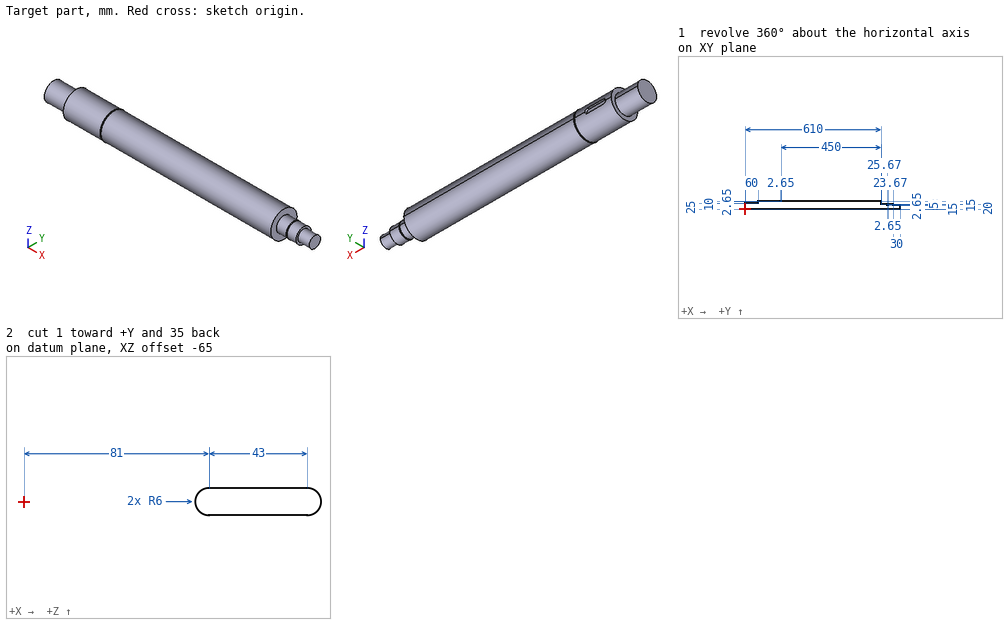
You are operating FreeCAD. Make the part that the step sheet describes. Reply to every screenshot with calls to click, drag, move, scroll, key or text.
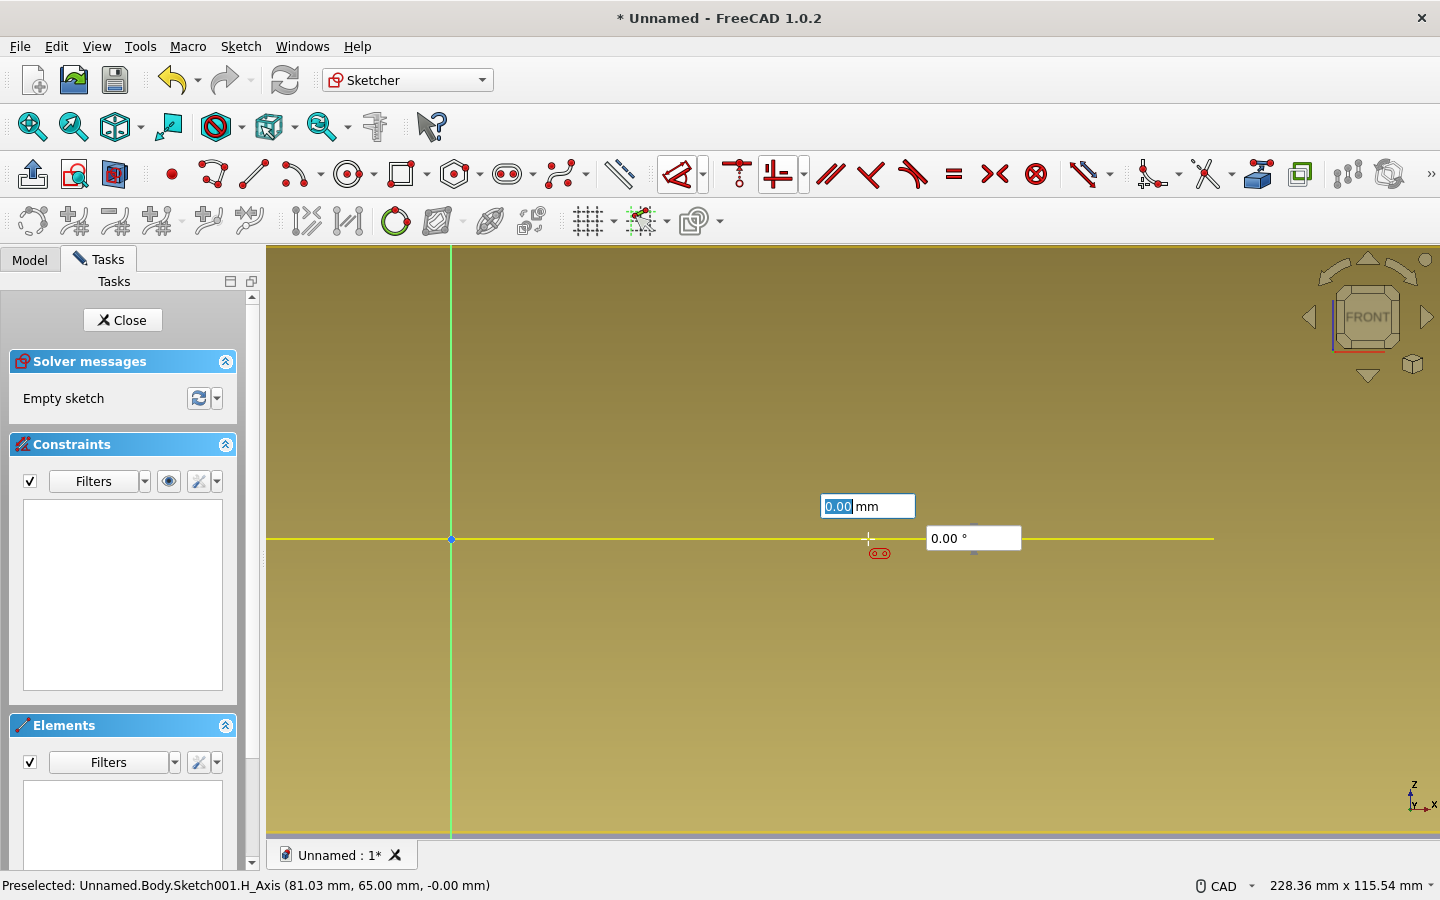
click(1089, 530)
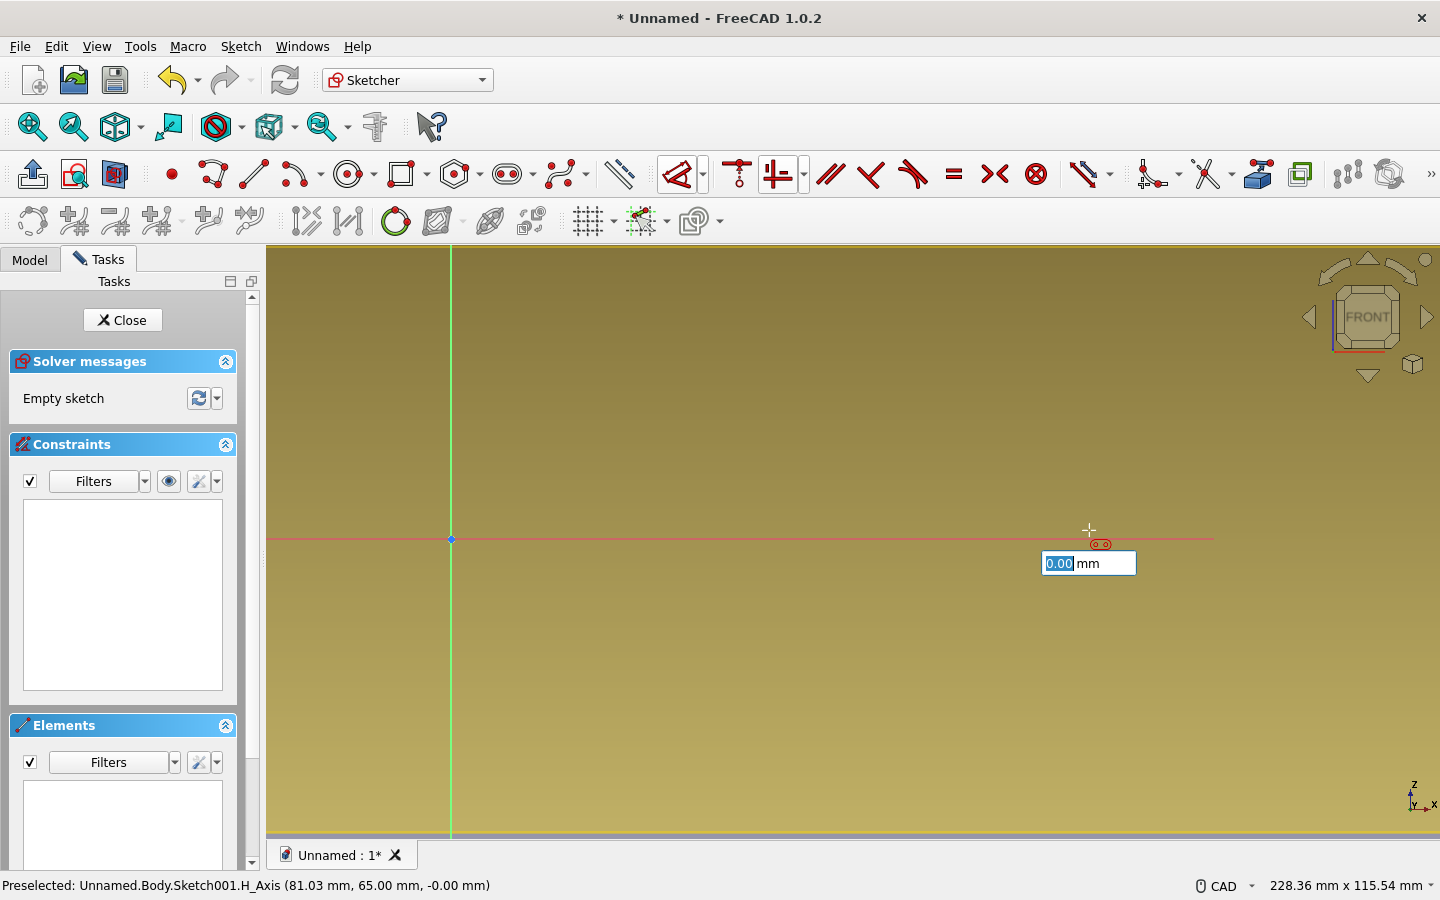
click(978, 570)
key(Escape)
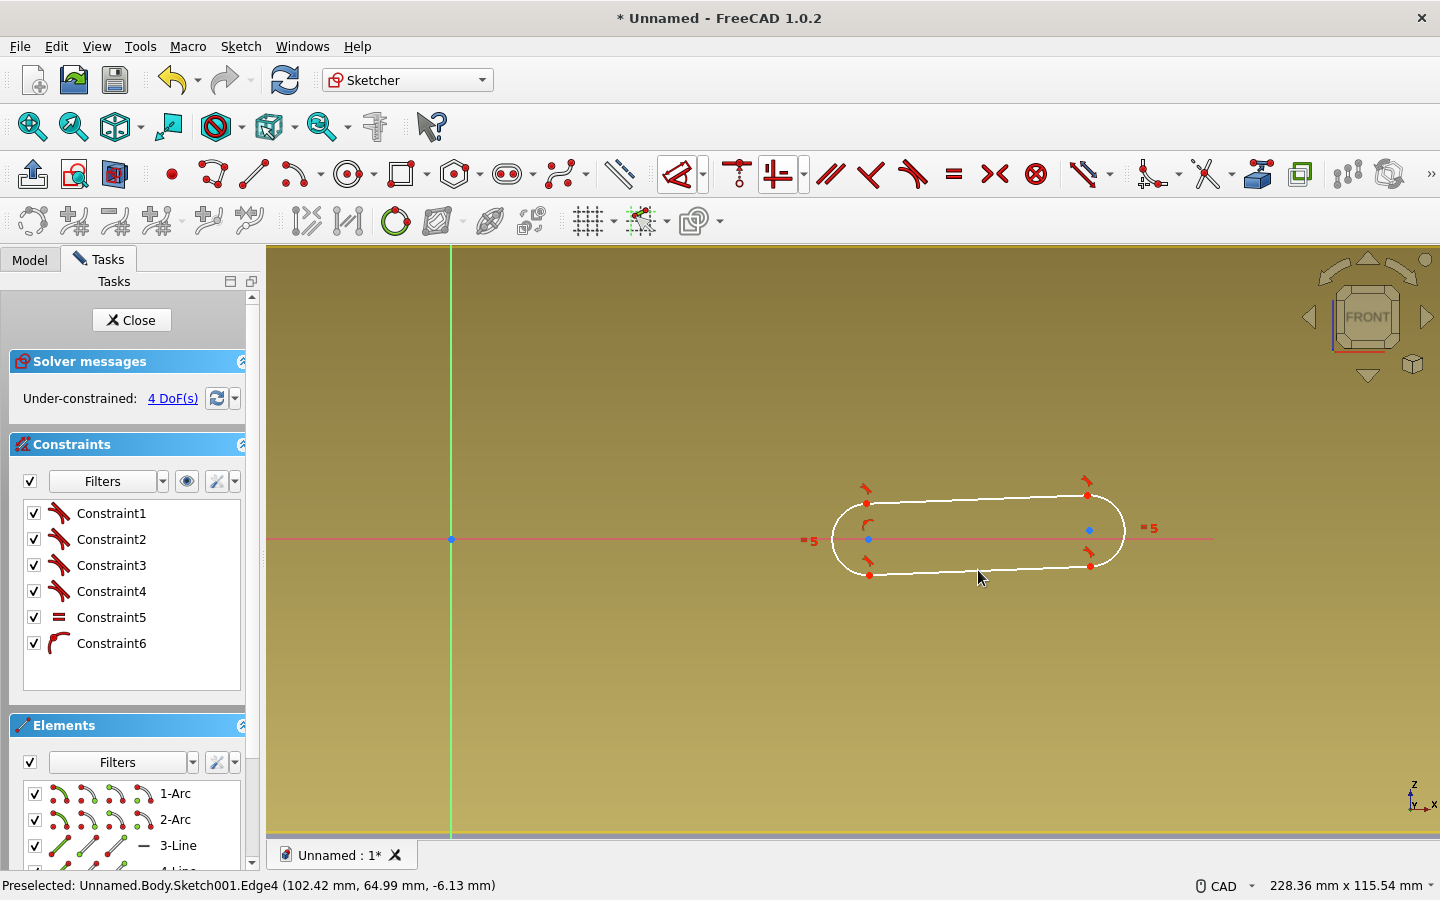
click(933, 501)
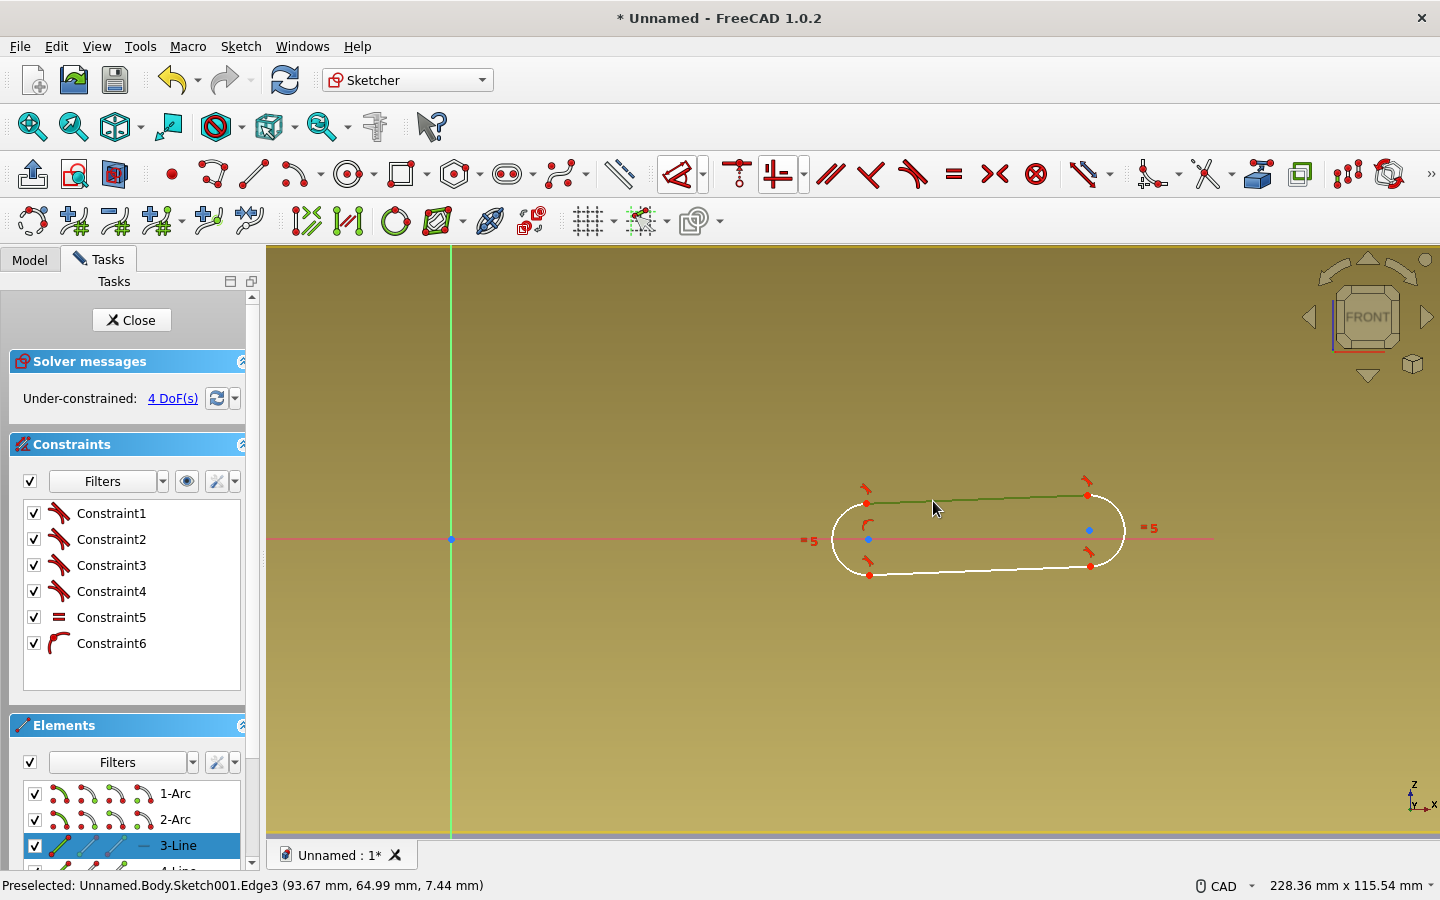
click(804, 174)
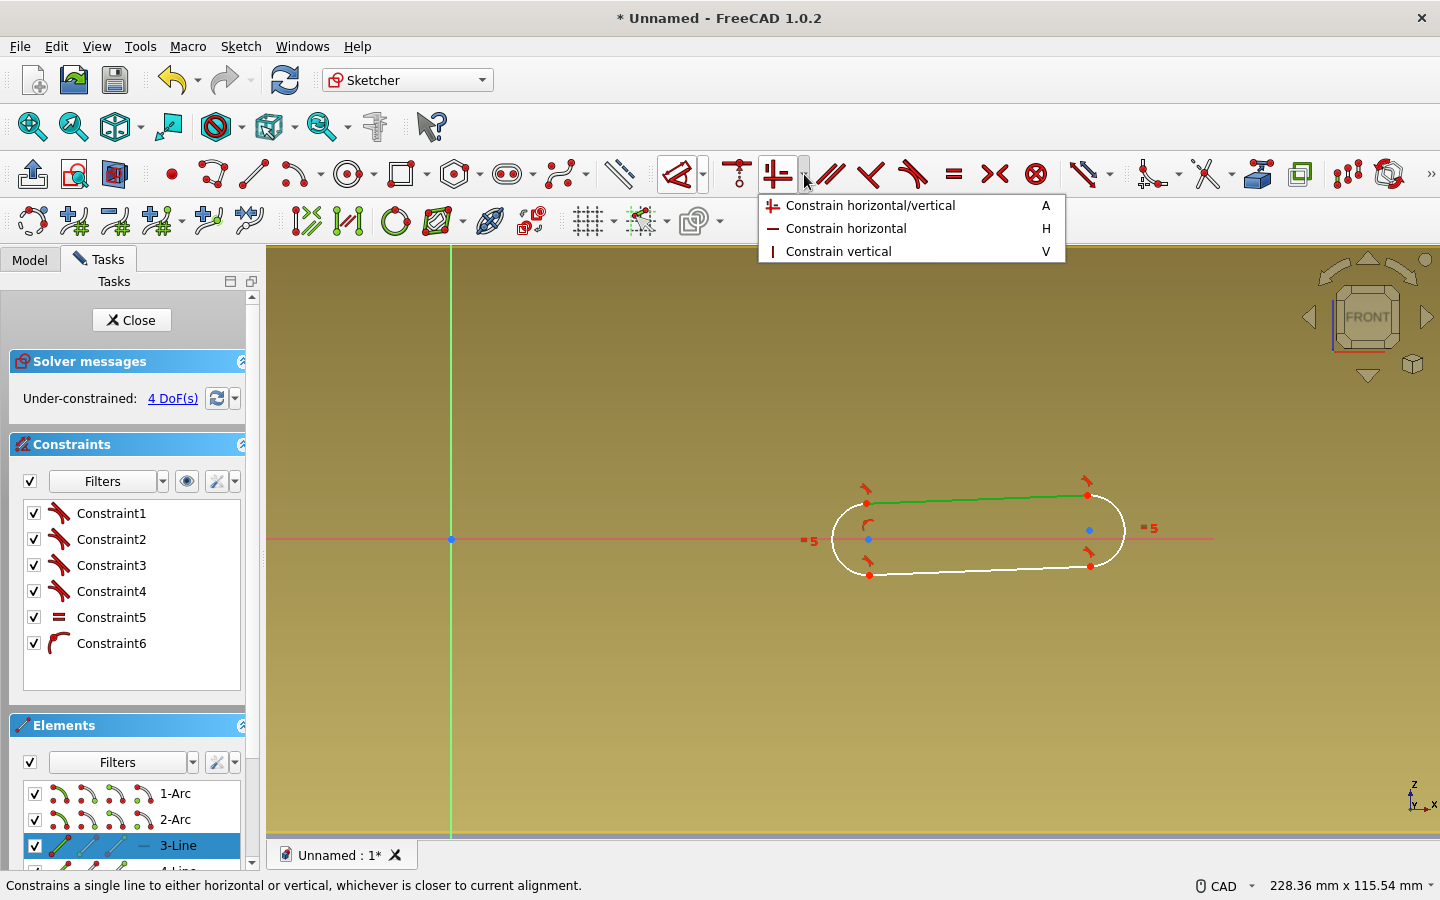
click(912, 228)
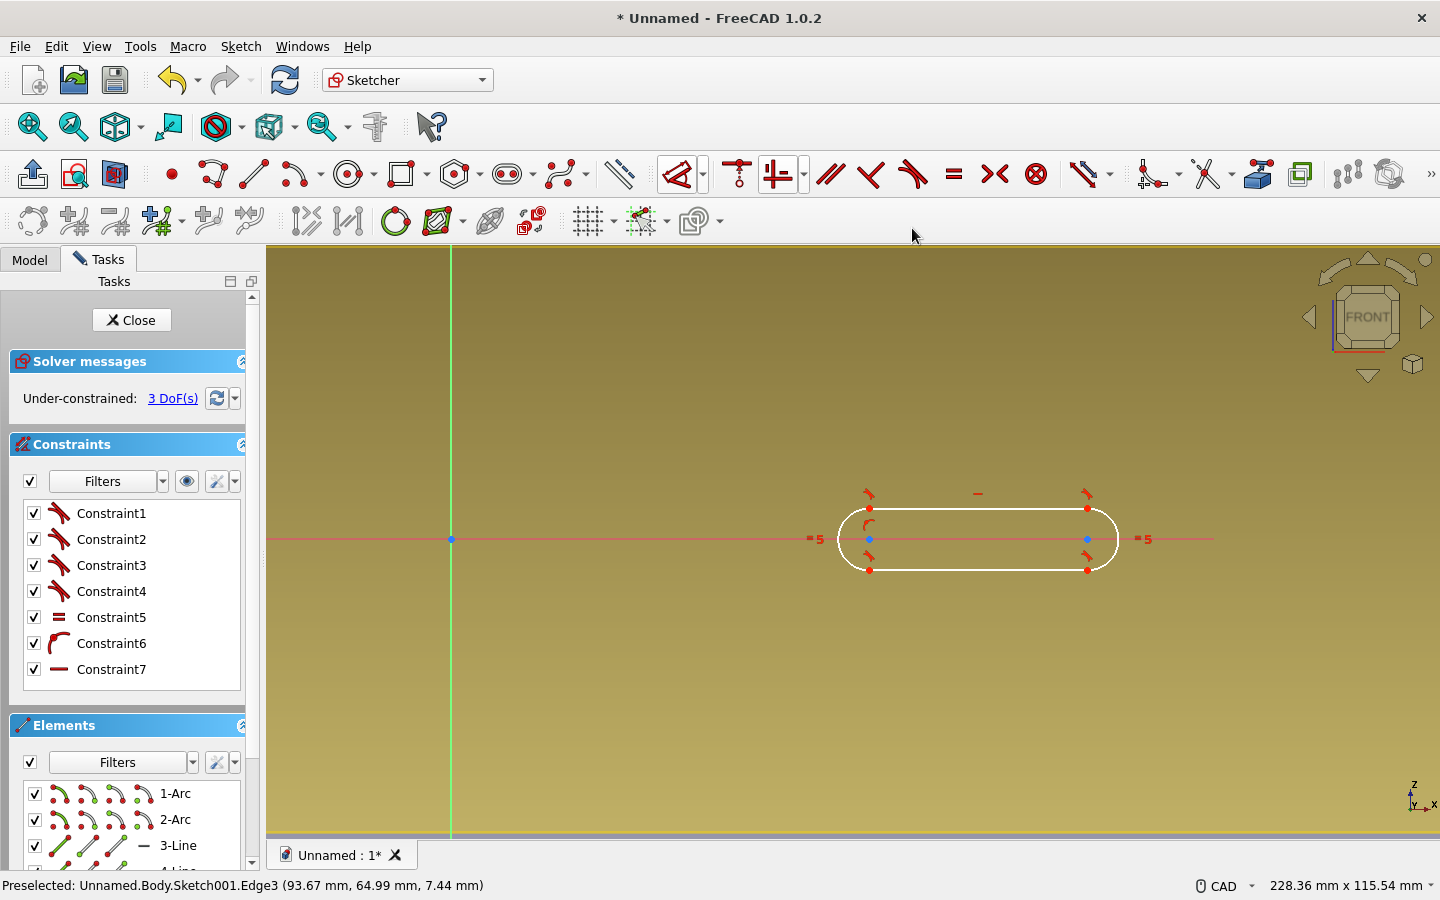
scroll(844, 521, up, 2)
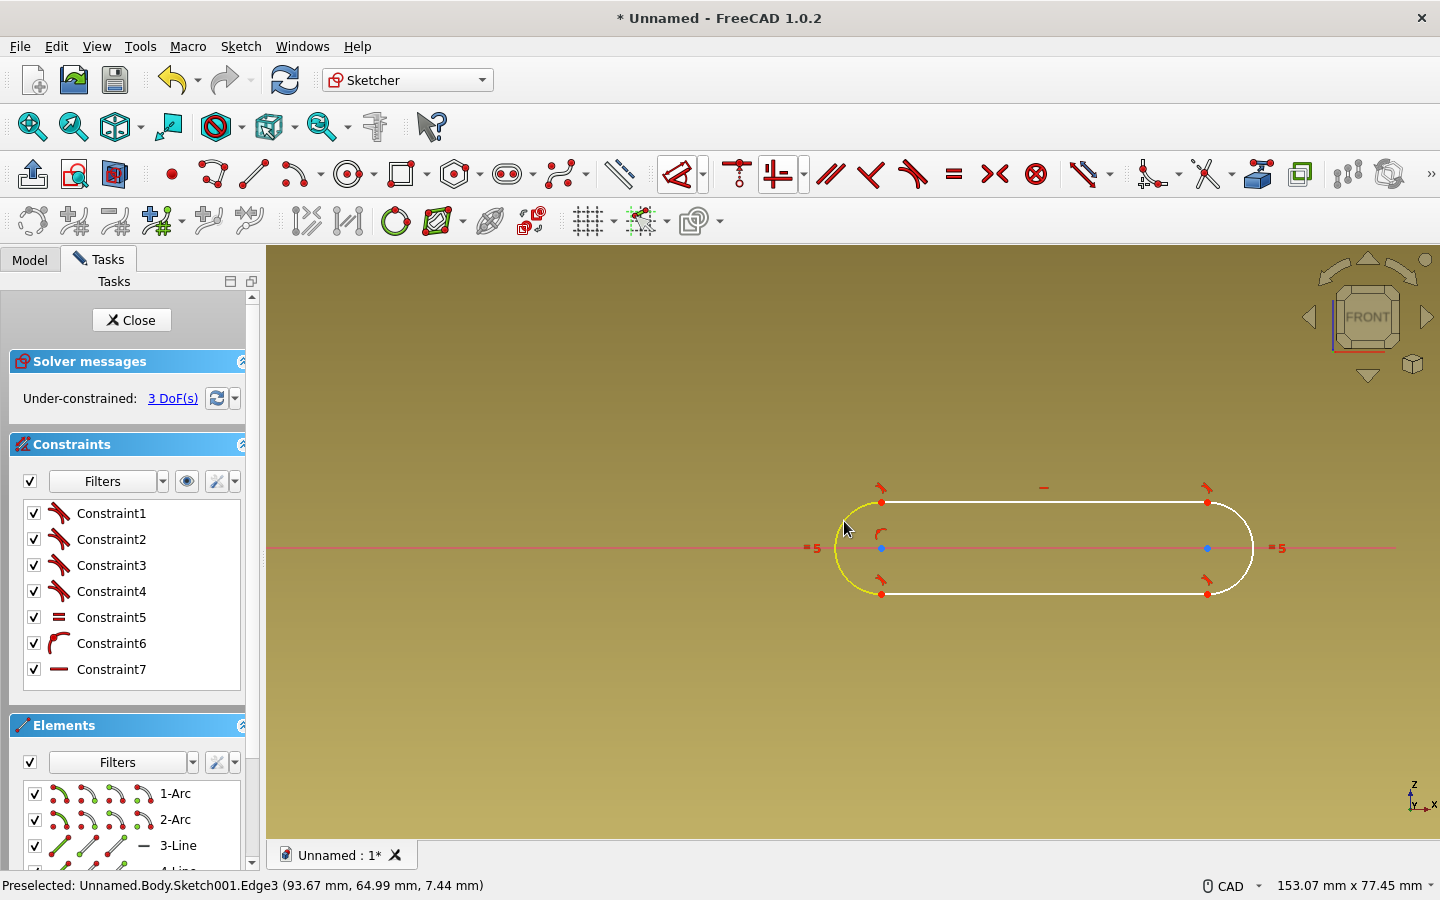
click(844, 521)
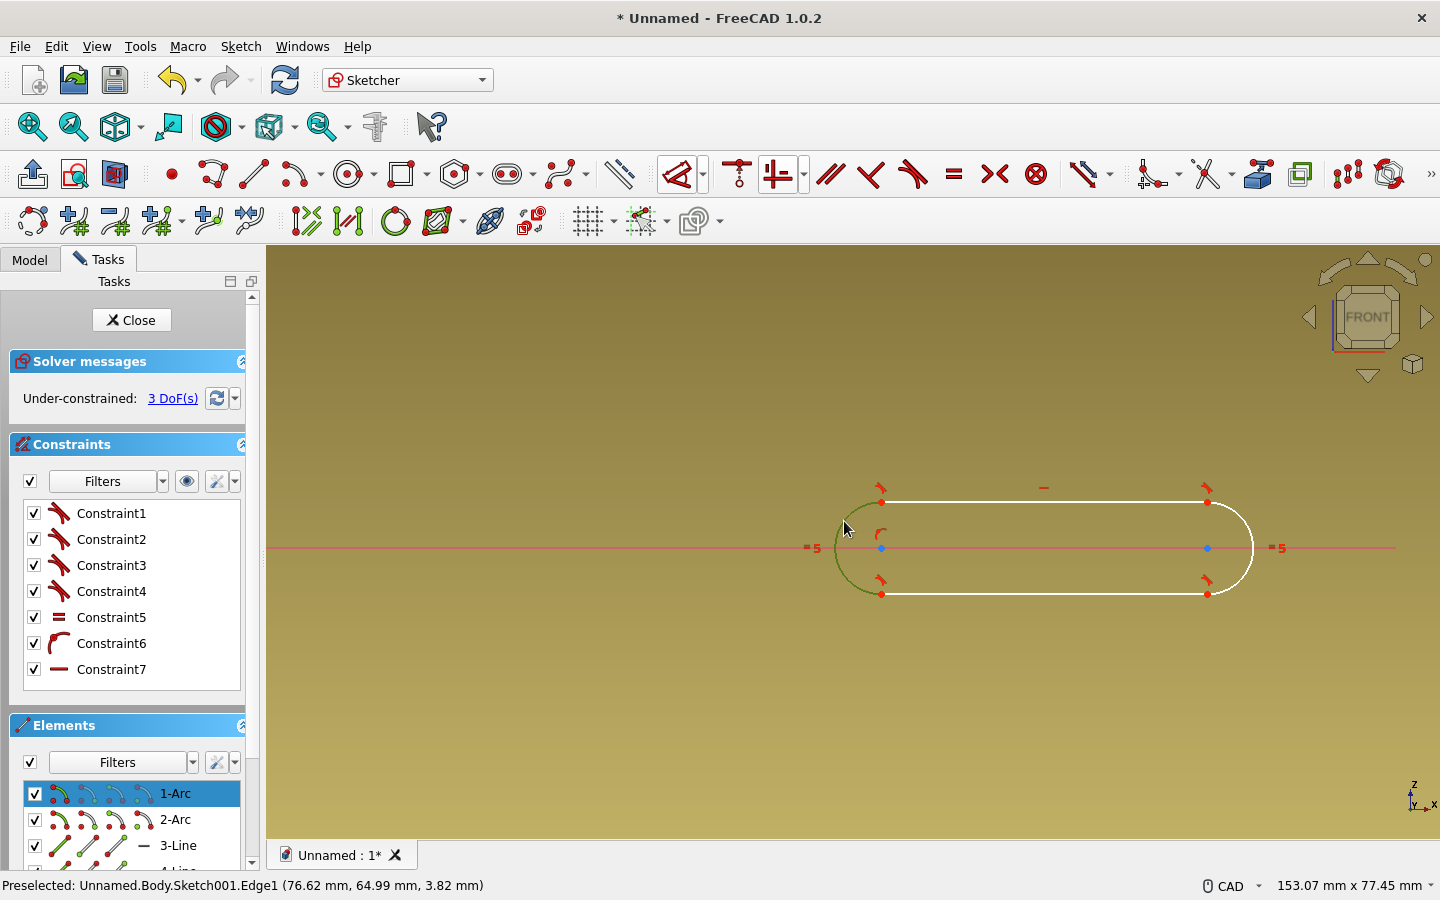
click(702, 174)